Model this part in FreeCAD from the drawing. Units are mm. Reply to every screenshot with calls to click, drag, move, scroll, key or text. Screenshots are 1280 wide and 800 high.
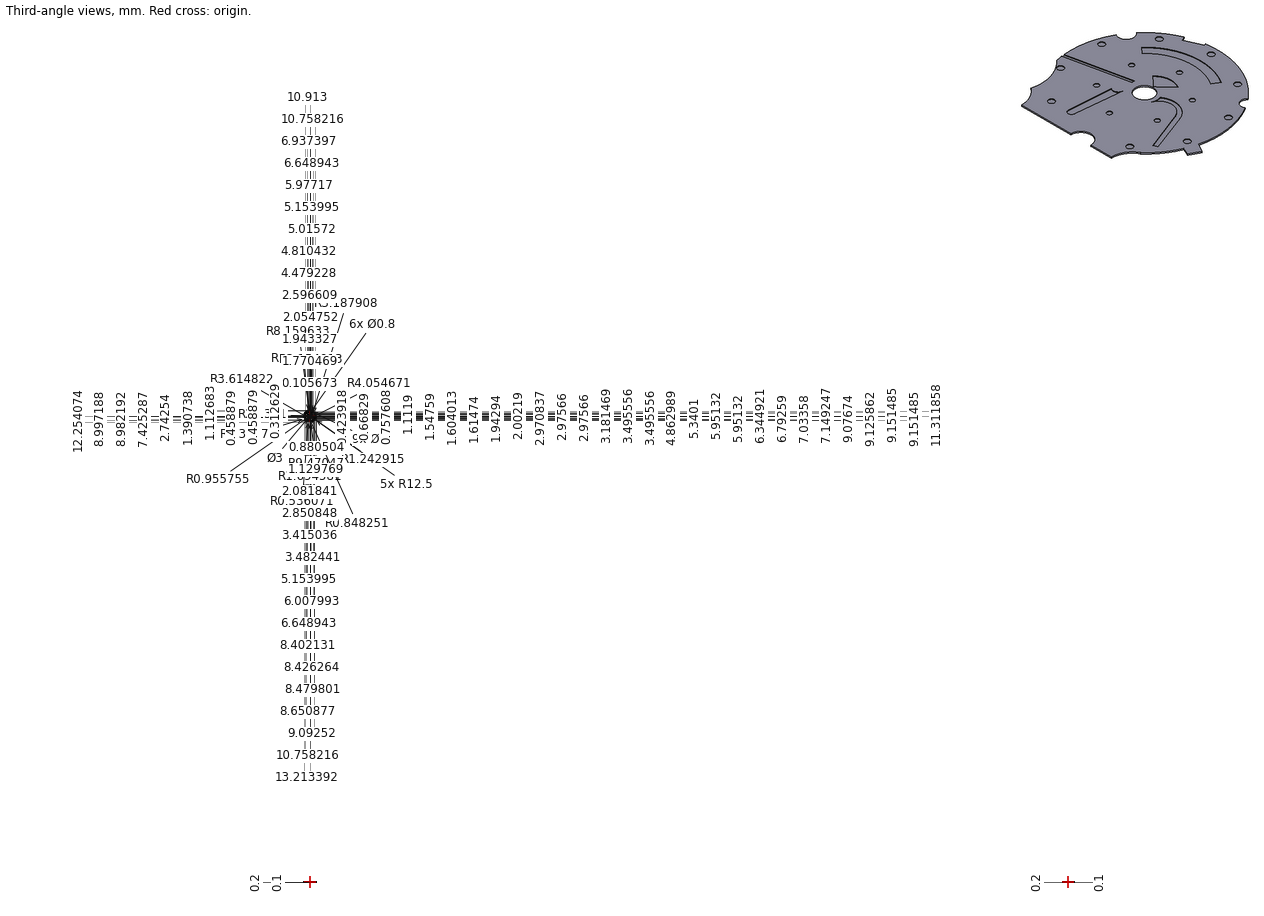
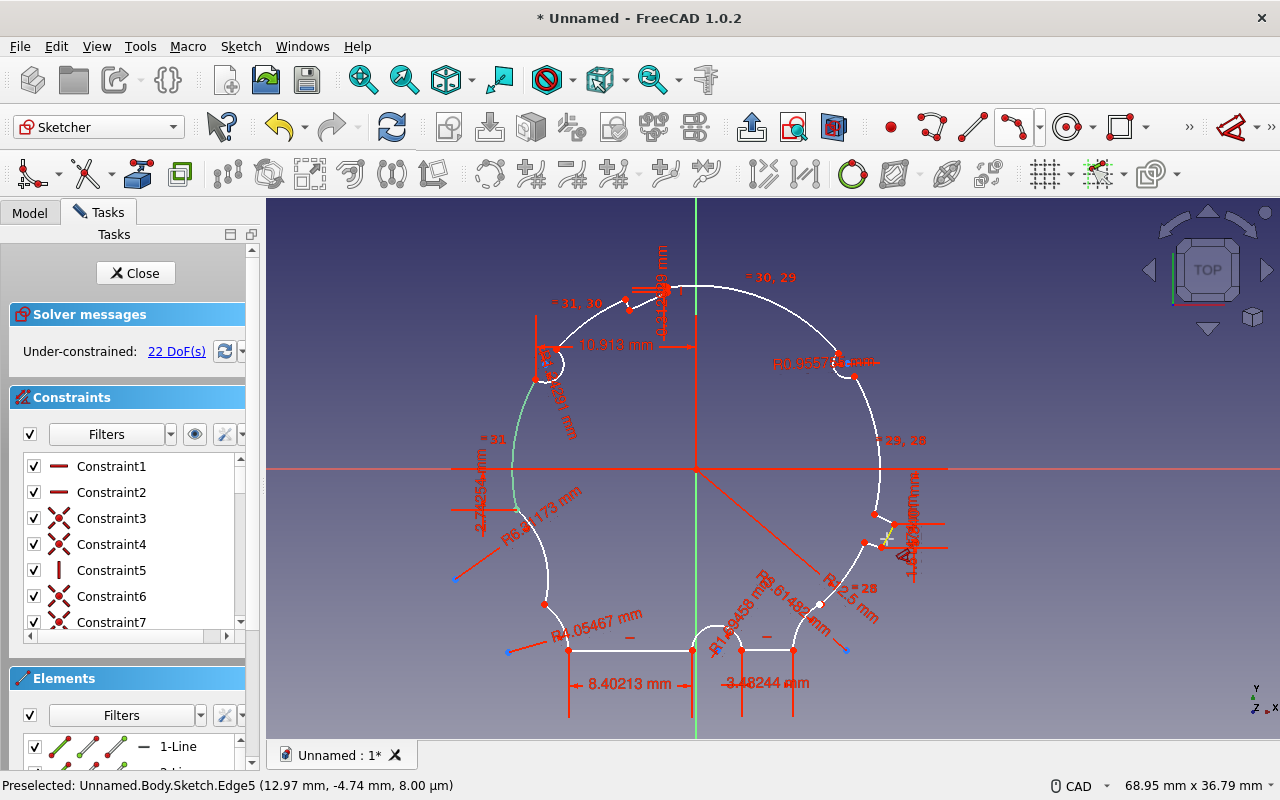
click(569, 651)
click(632, 435)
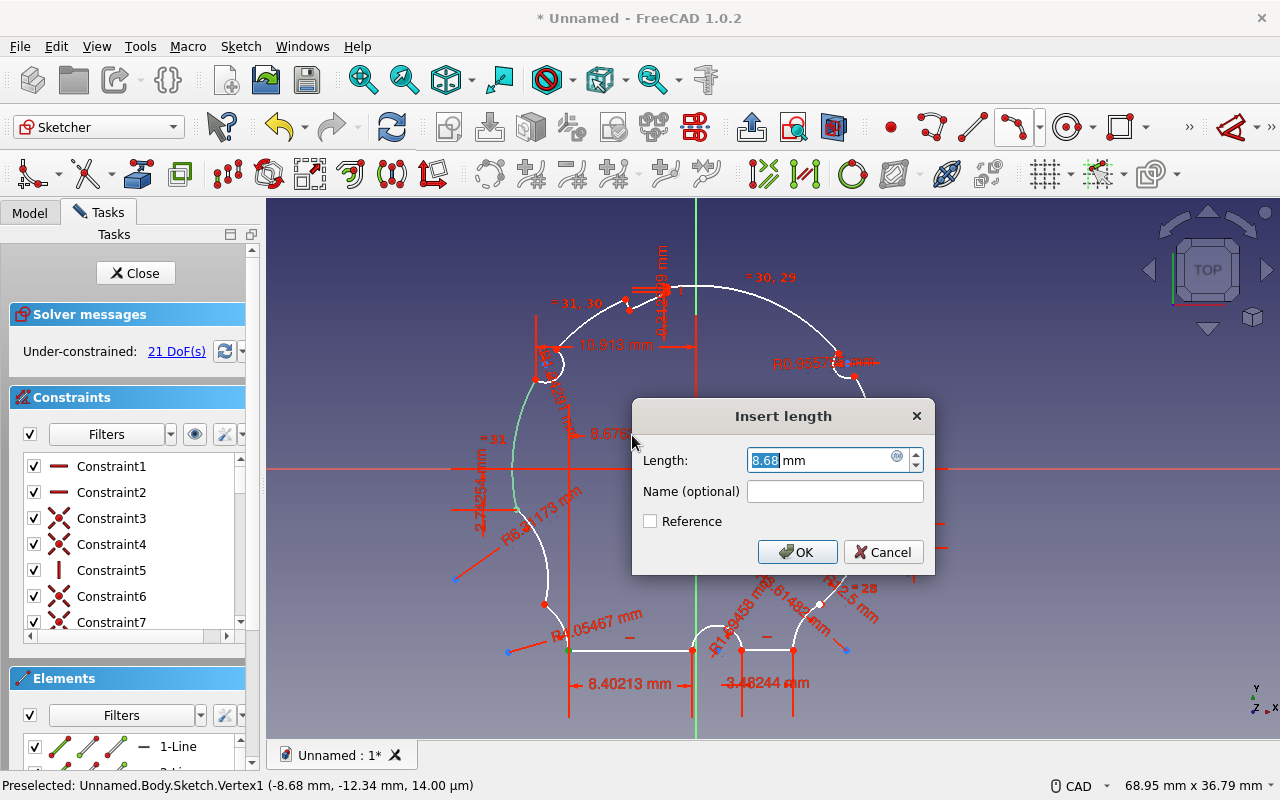
text(8.650877)
key(Return)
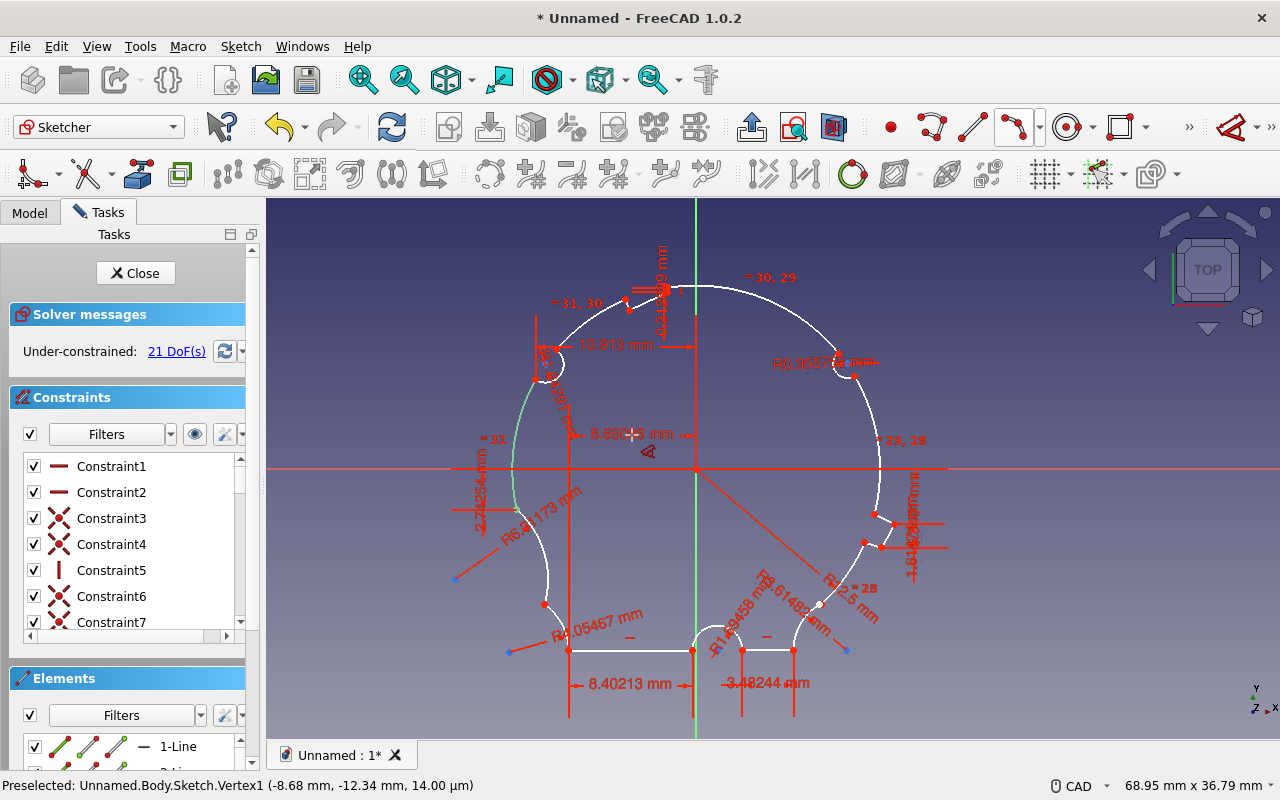
scroll(820, 604, up, 11)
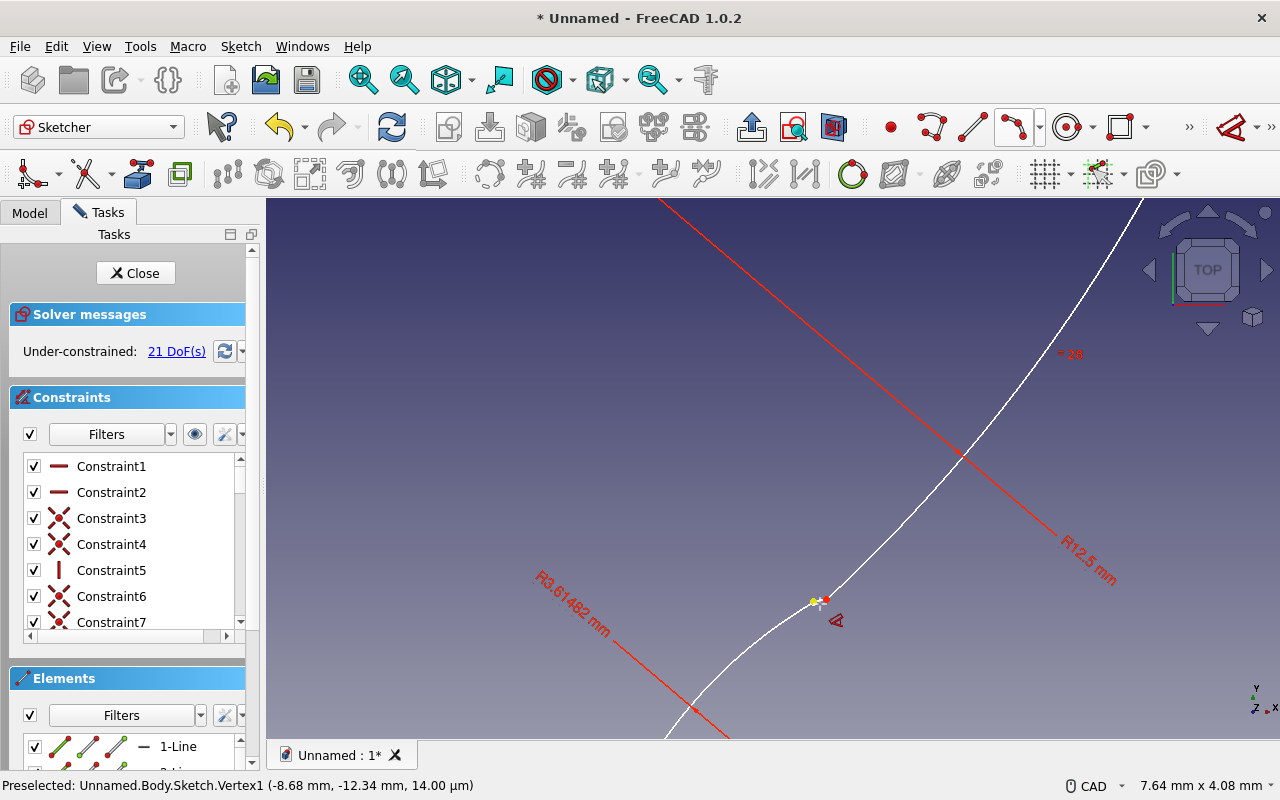
click(814, 601)
click(554, 635)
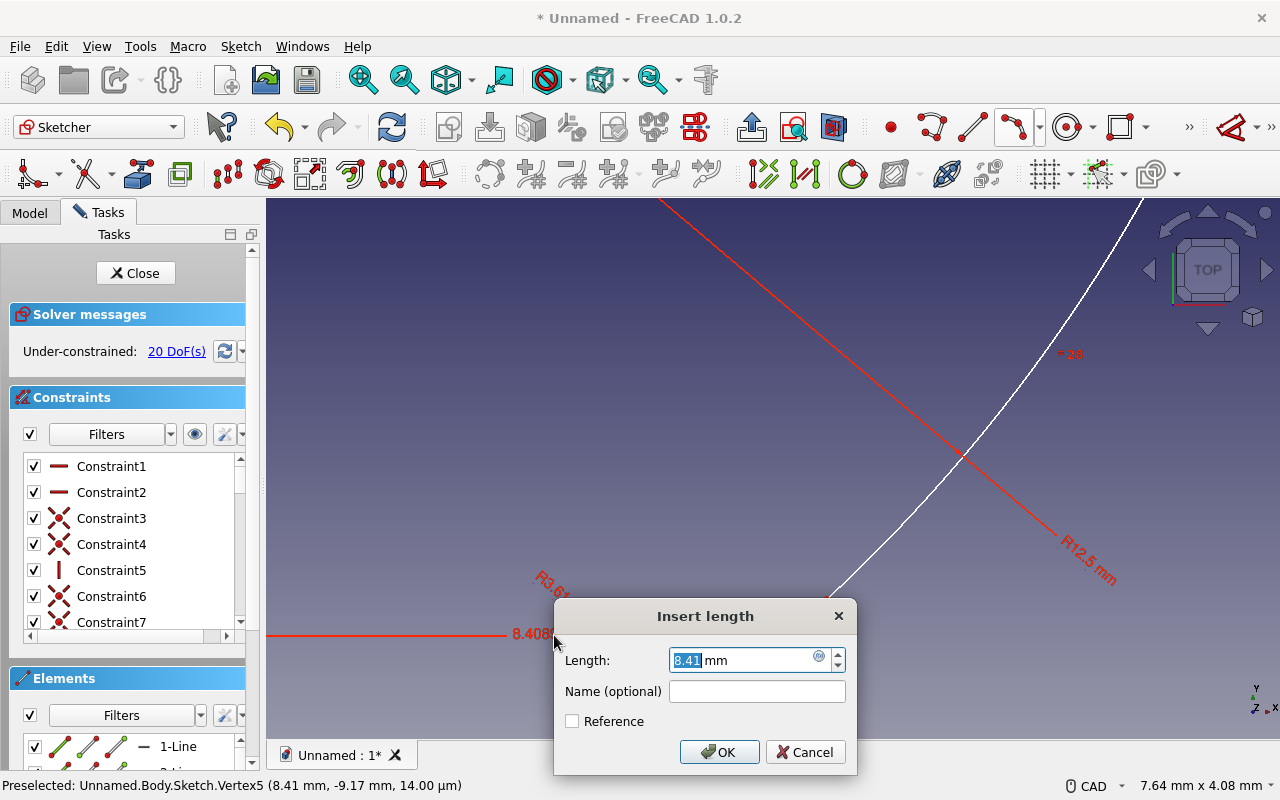
text(8.426264)
key(Return)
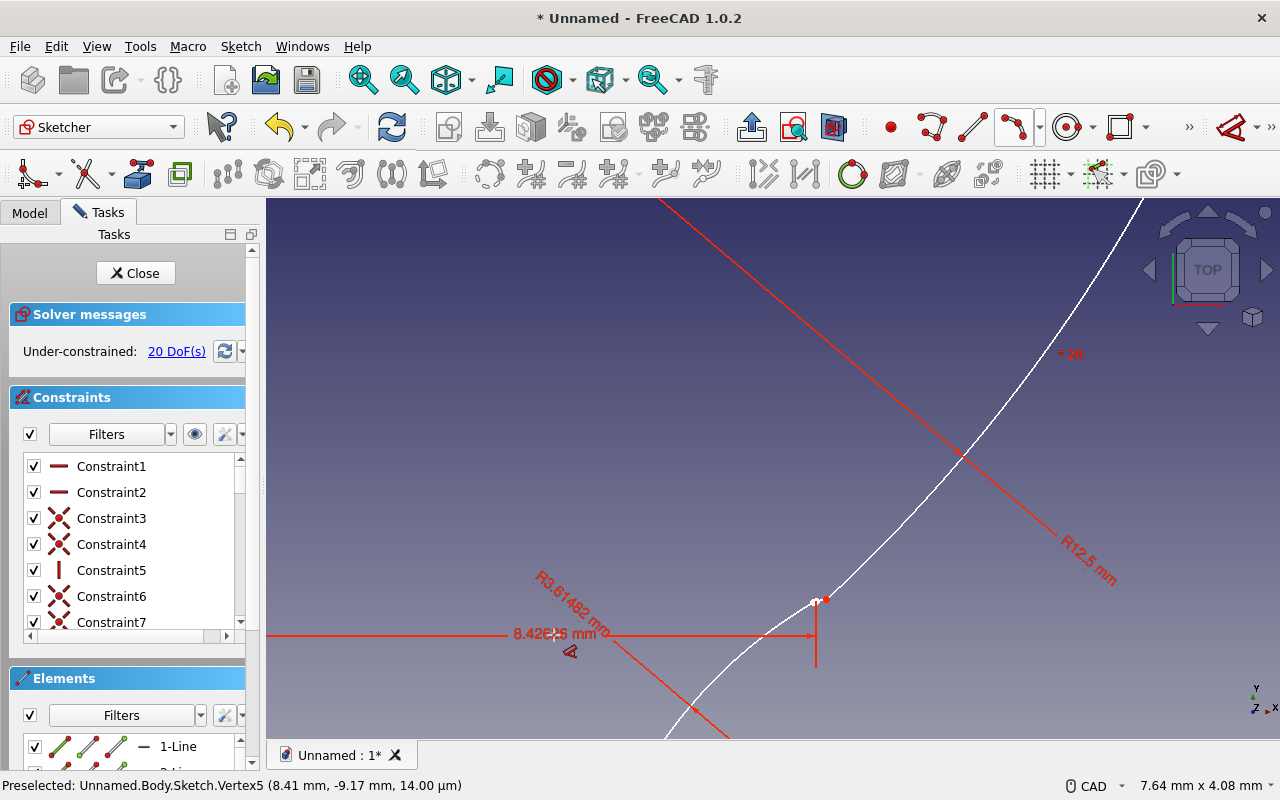
click(816, 601)
click(850, 414)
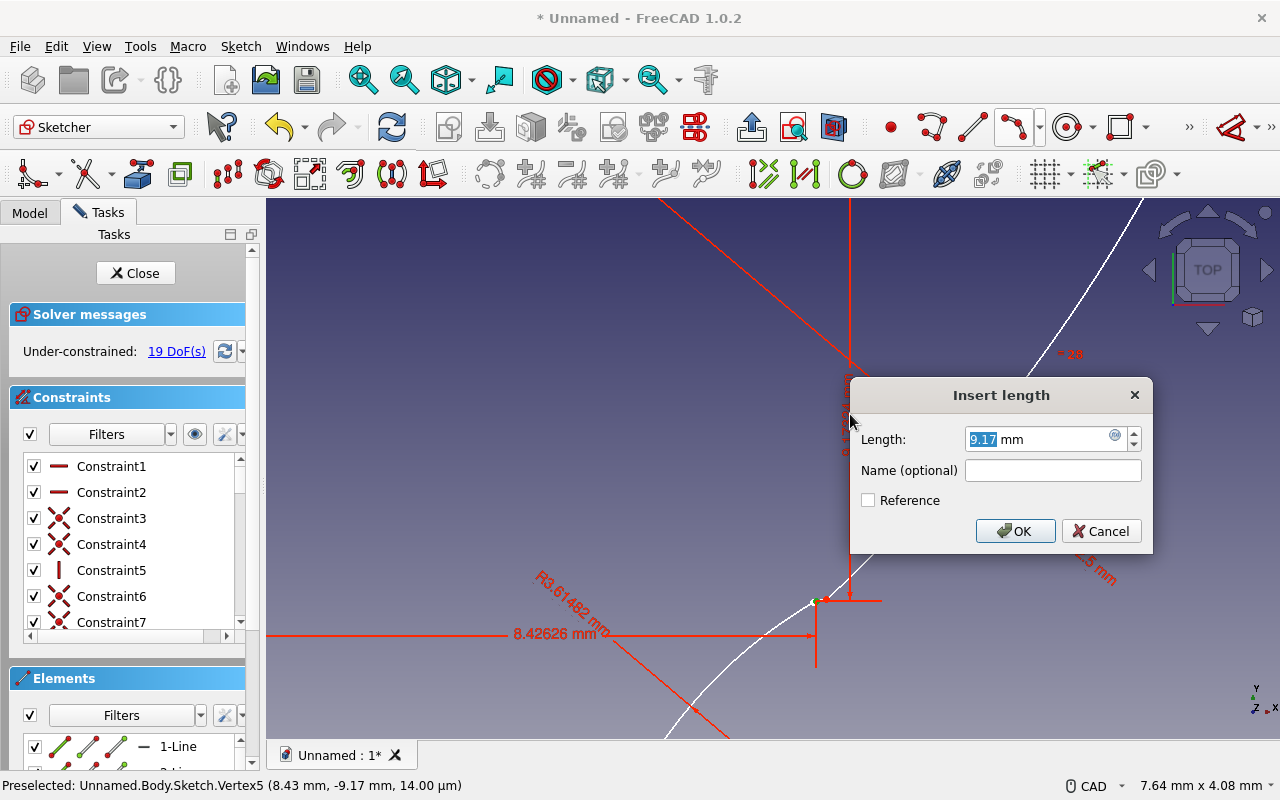
text(9.125862)
key(Return)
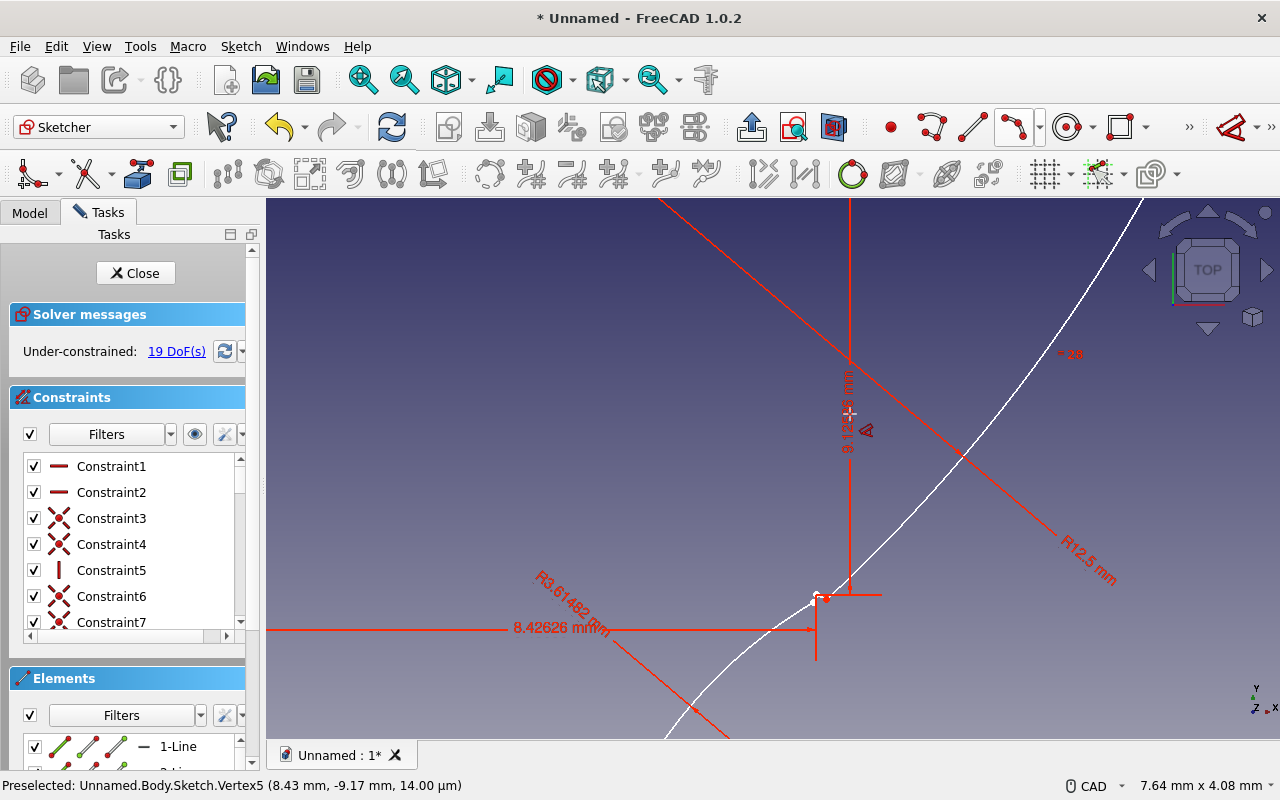
click(827, 599)
click(438, 633)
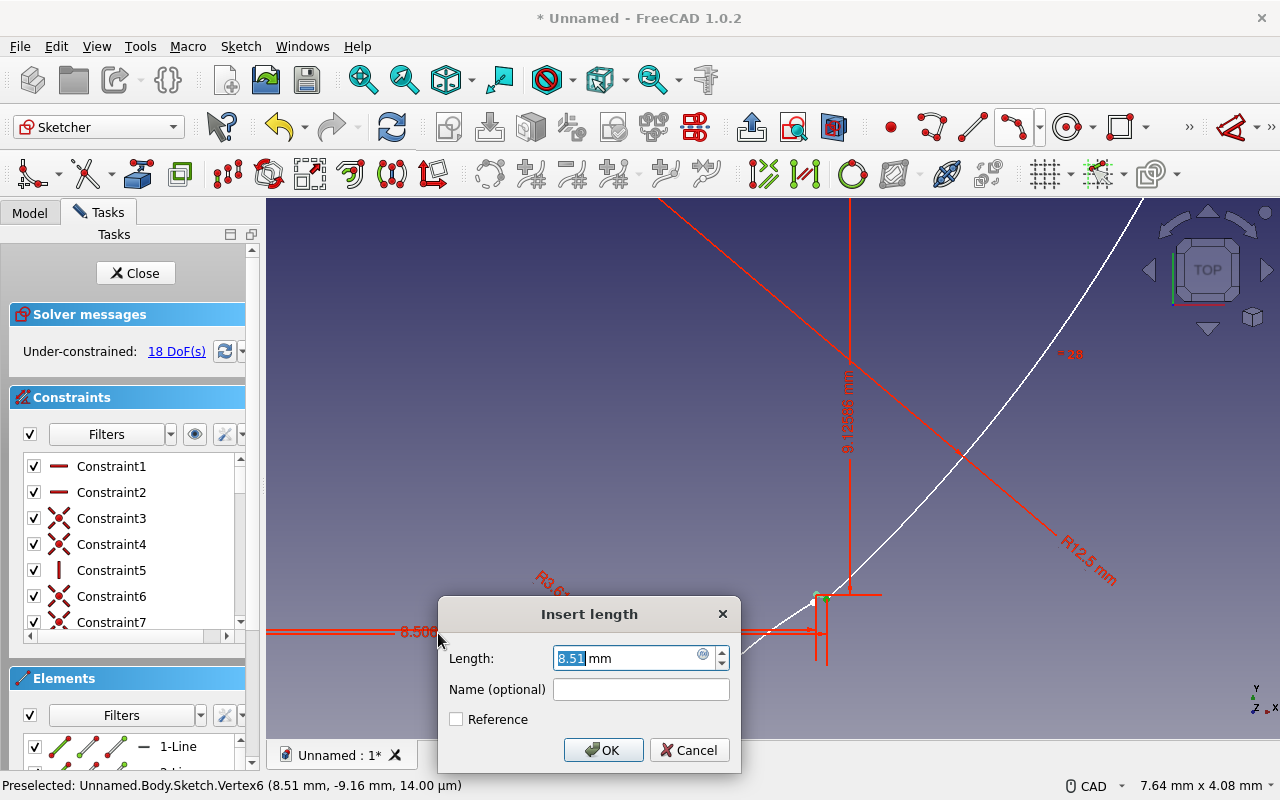
text(8.479801)
key(Return)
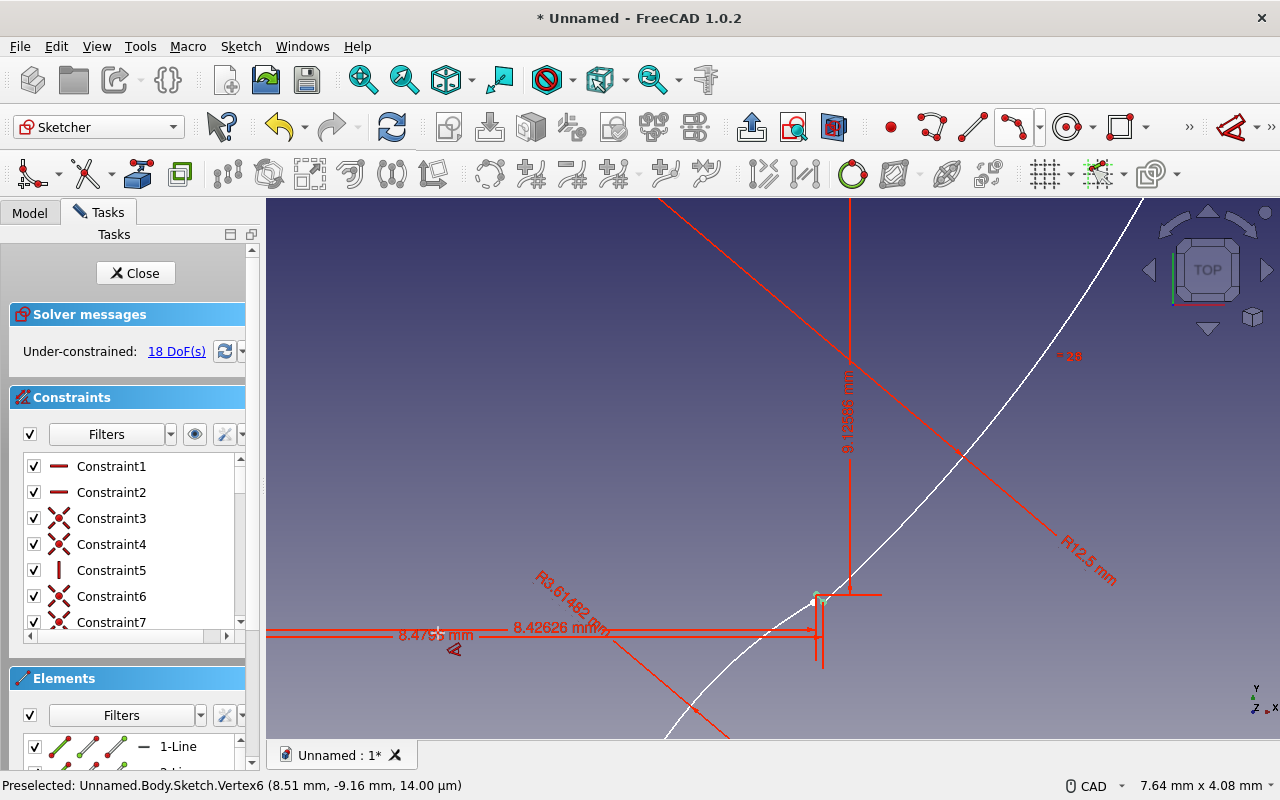
scroll(820, 604, down, 11)